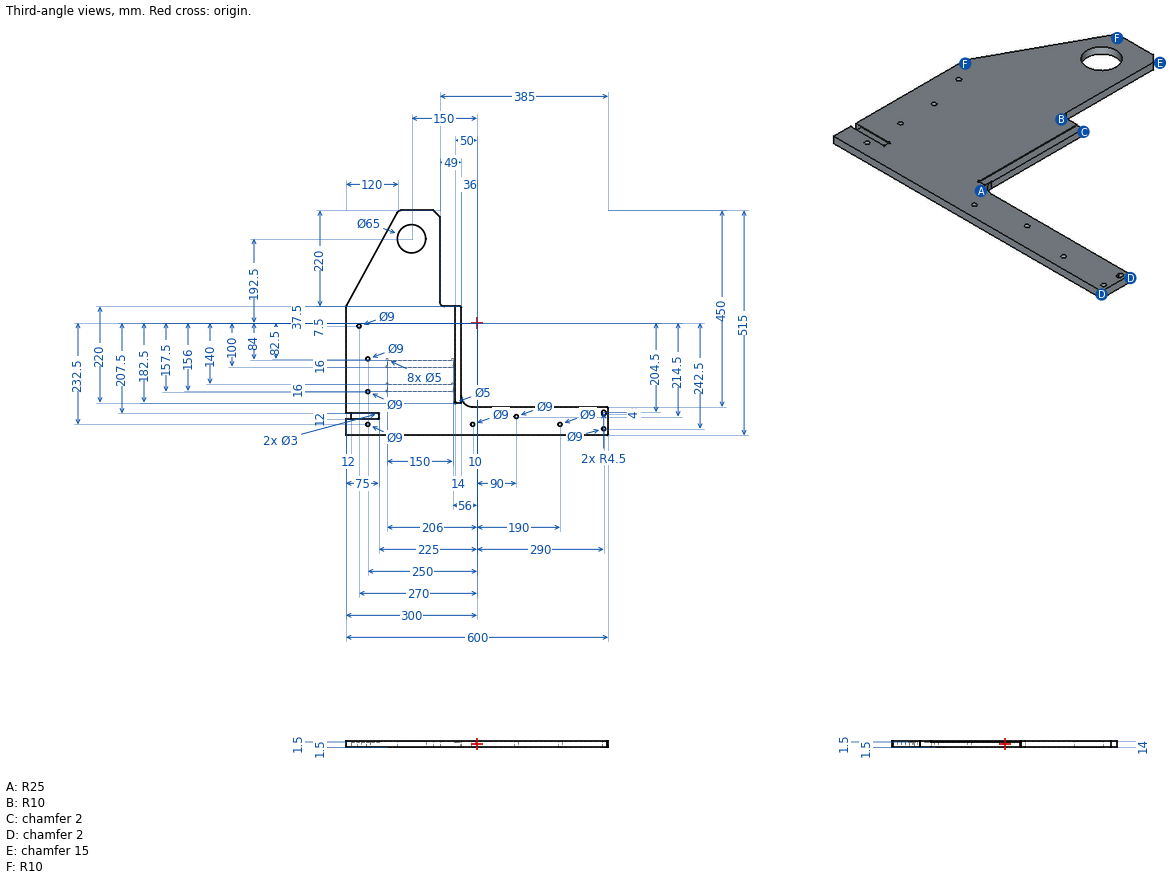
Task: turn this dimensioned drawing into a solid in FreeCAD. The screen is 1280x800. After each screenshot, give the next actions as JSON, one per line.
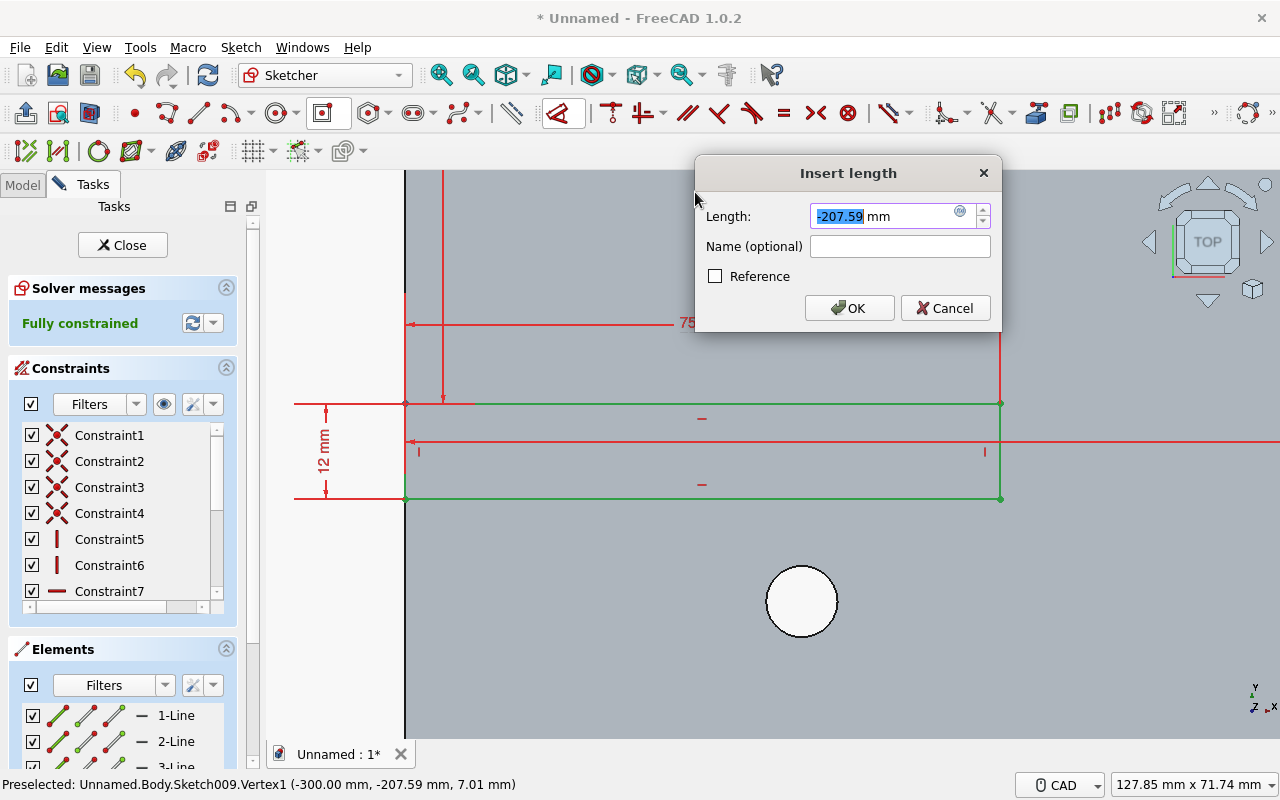
{"action": "type", "text": "-207.5"}
{"action": "key", "text": "Return"}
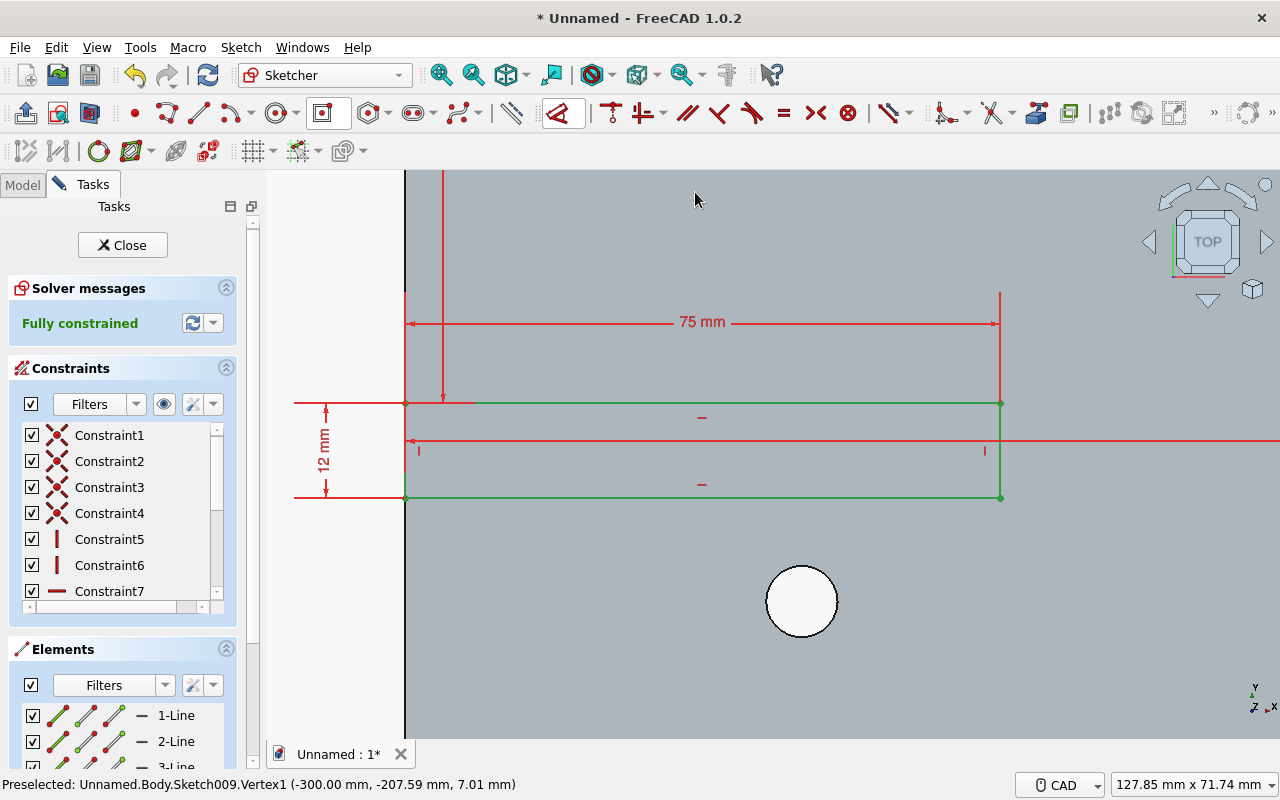
{"action": "left_click", "coordinate": [123, 245]}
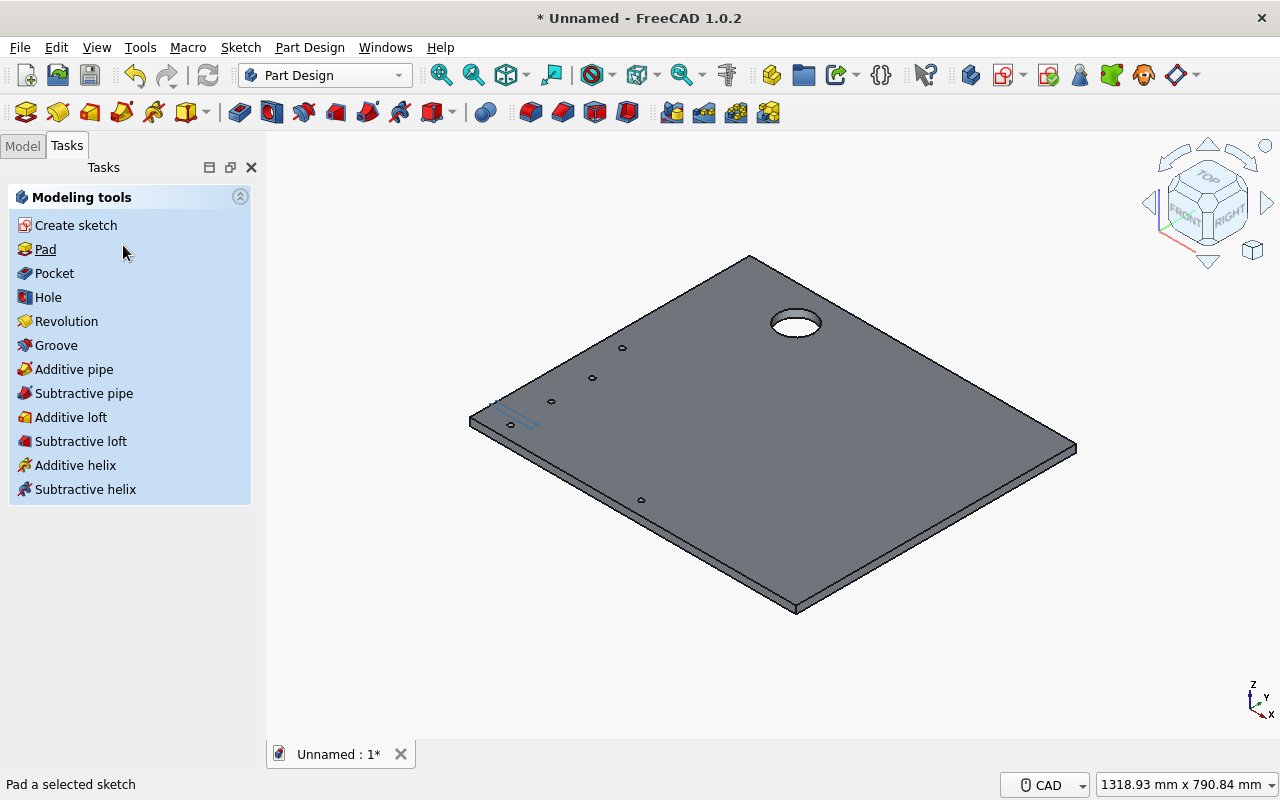
{"action": "left_click", "coordinate": [240, 112]}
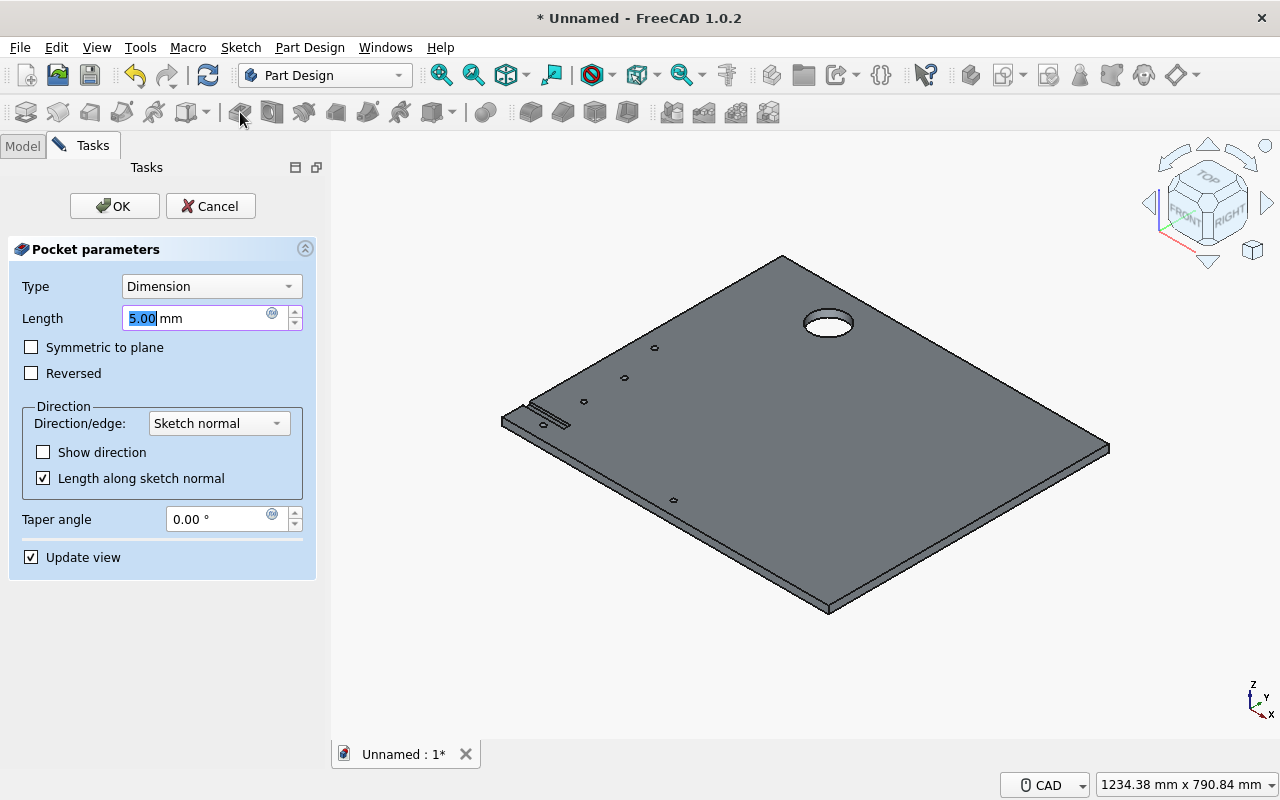
{"action": "type", "text": "1.5"}
{"action": "key", "text": "Tab"}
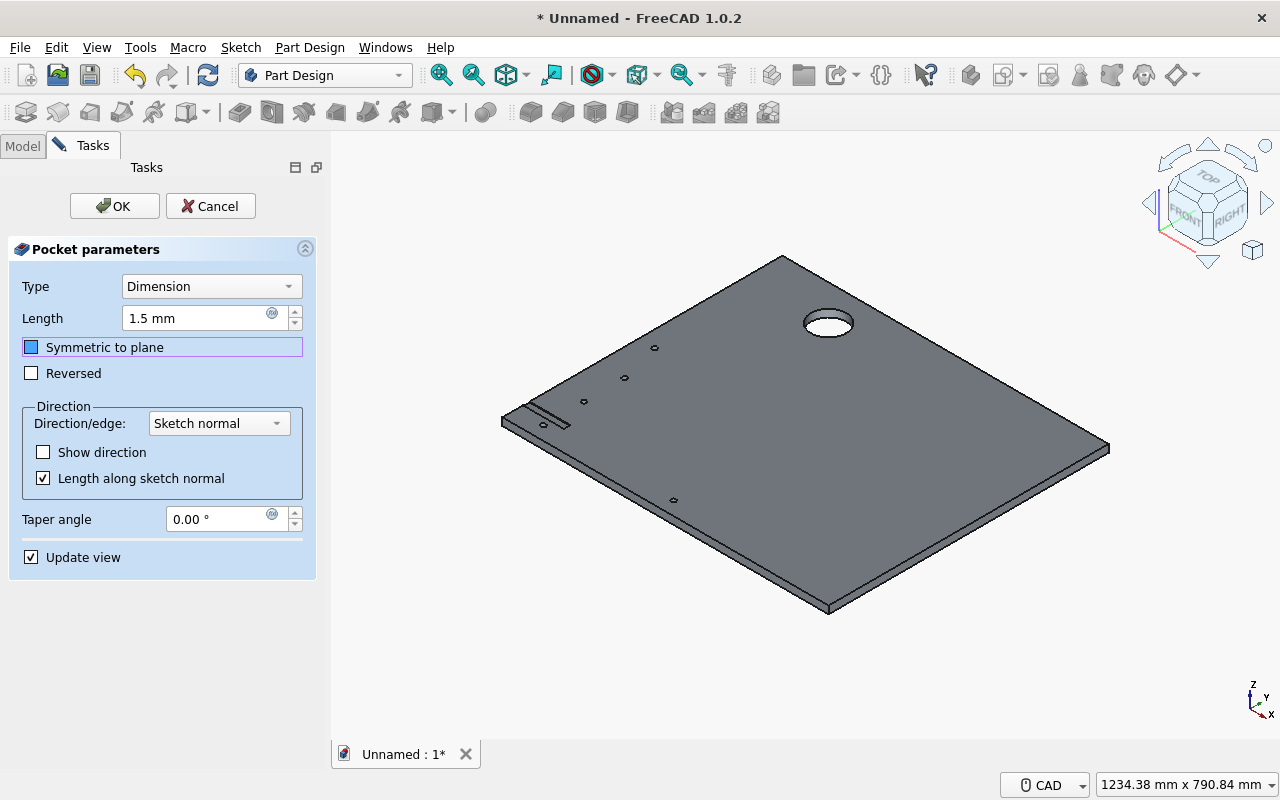
{"action": "left_click", "coordinate": [115, 206]}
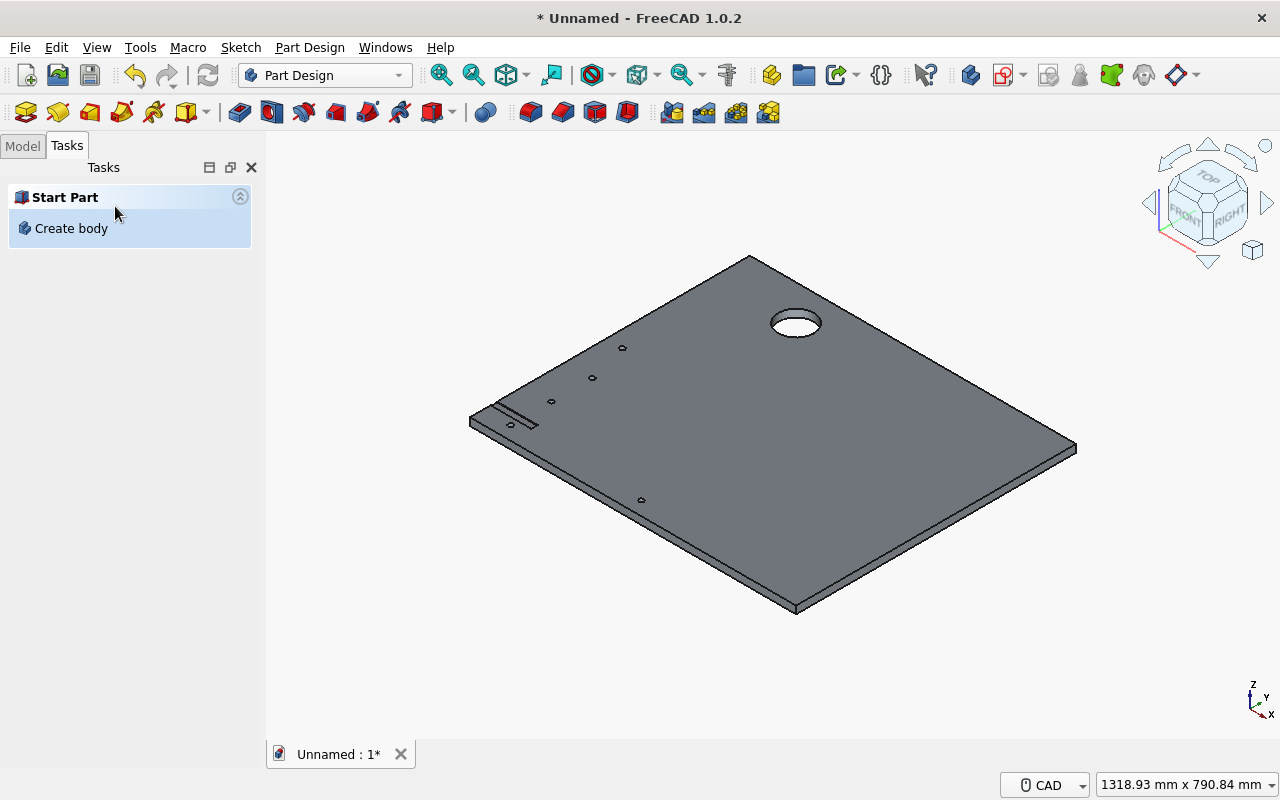
{"action": "left_click", "coordinate": [820, 457]}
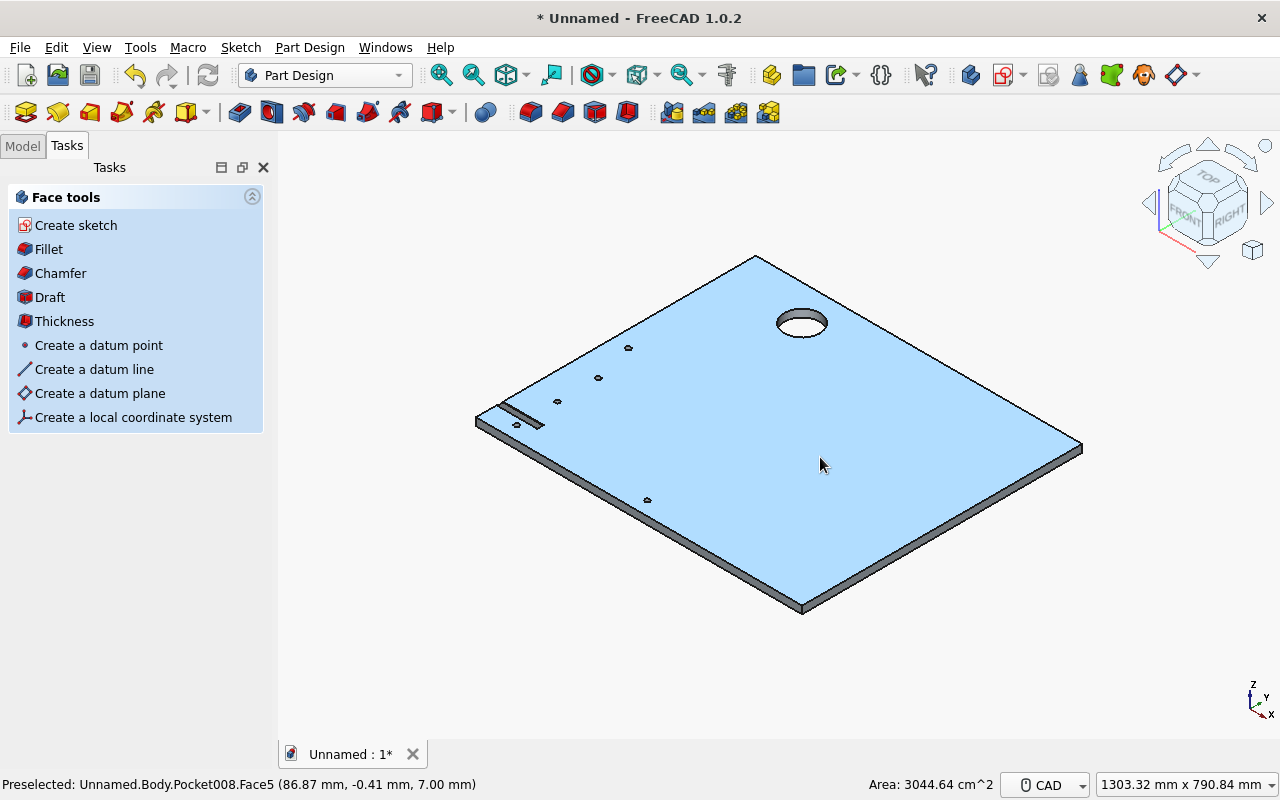
{"action": "left_click", "coordinate": [1004, 76]}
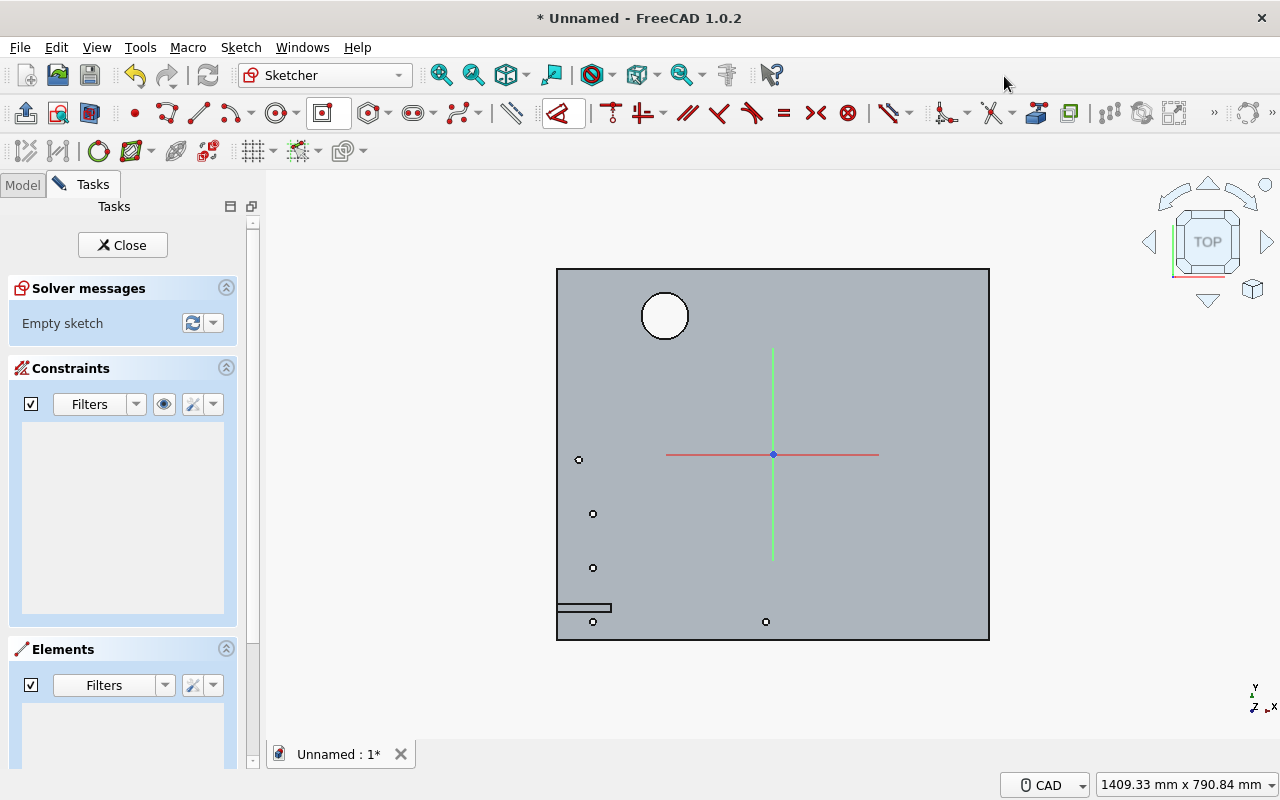
{"action": "scroll", "coordinate": [606, 616], "scroll_direction": "up", "scroll_amount": 15}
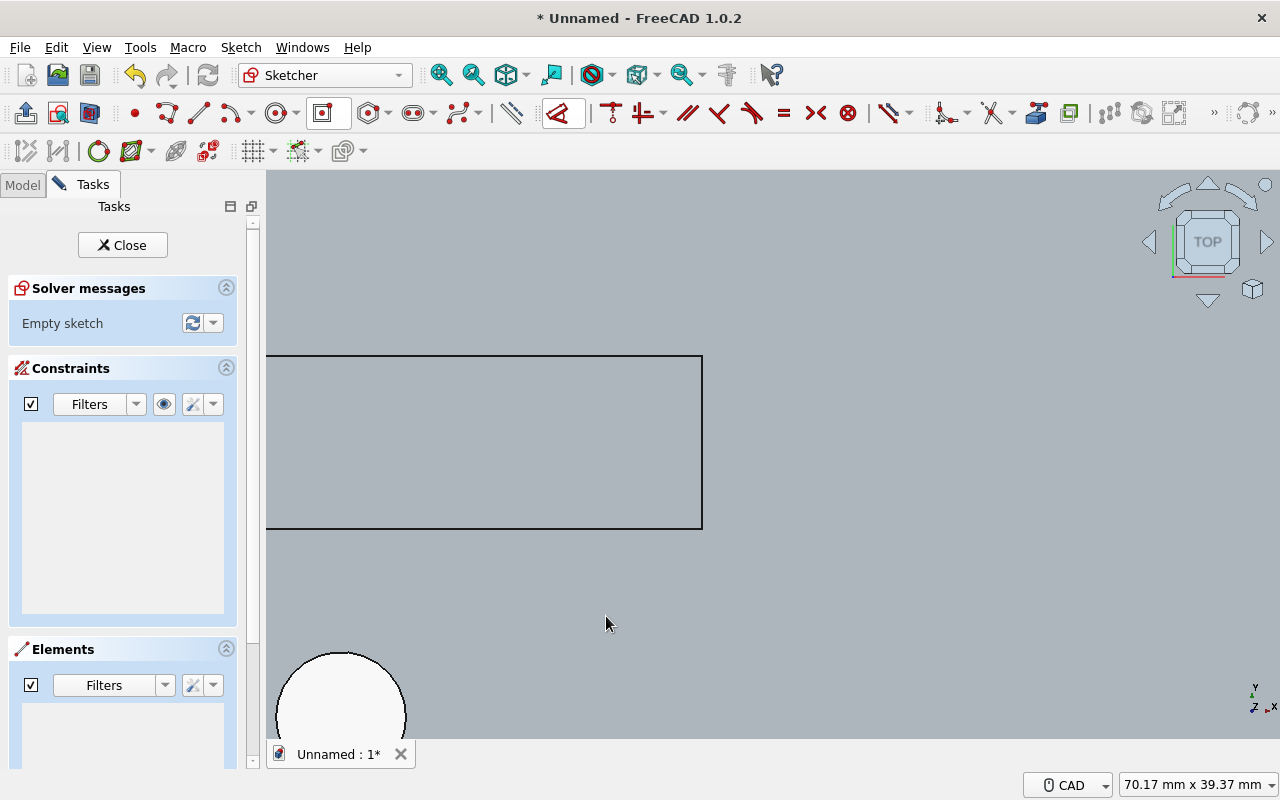
{"action": "scroll", "coordinate": [700, 428], "scroll_direction": "up", "scroll_amount": 3}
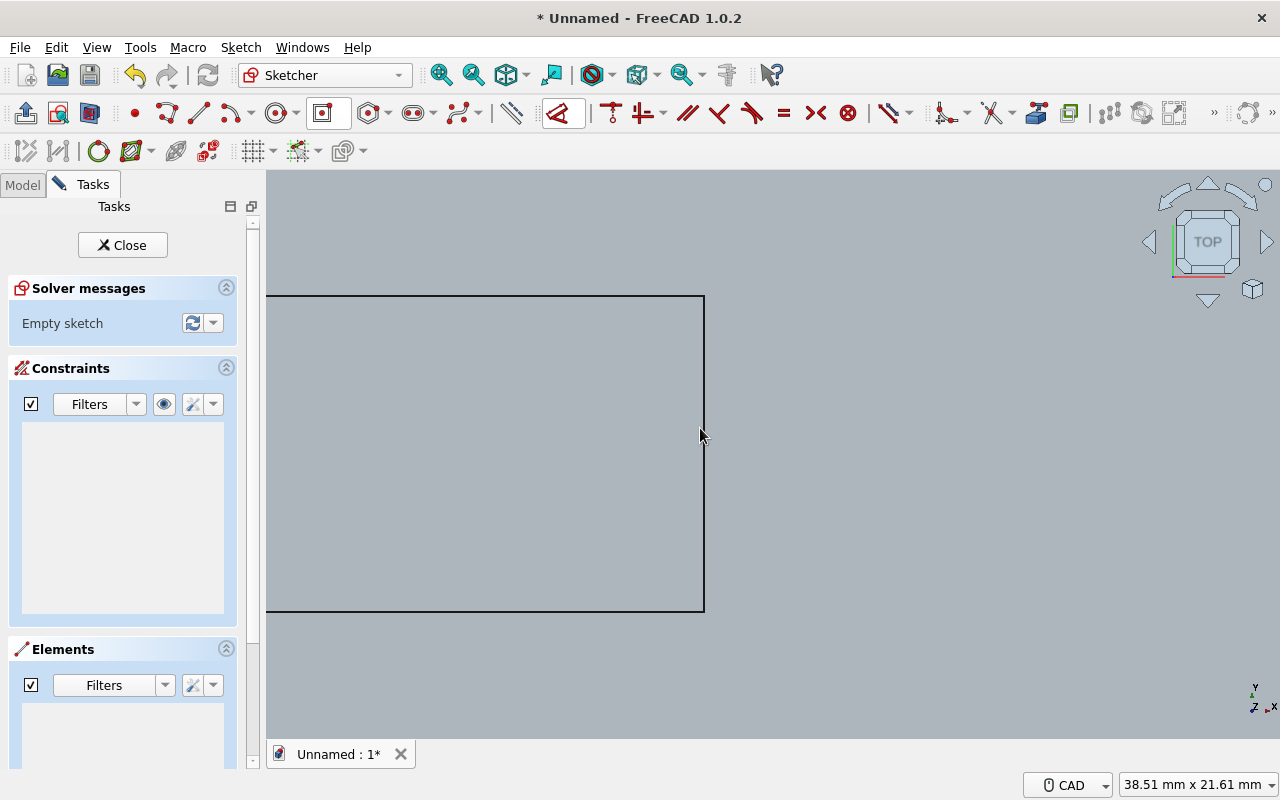
{"action": "left_click", "coordinate": [276, 114]}